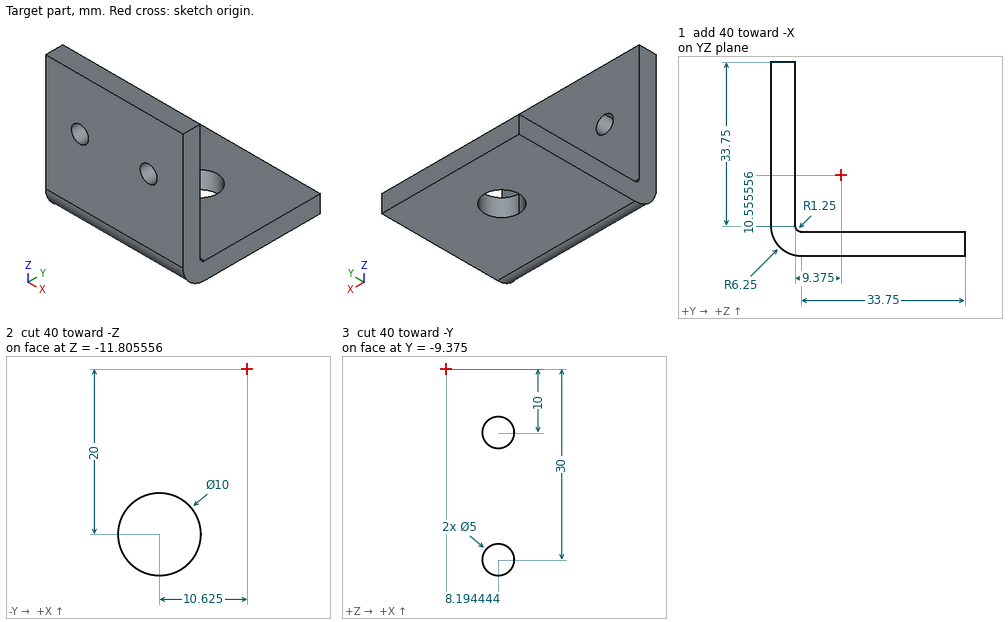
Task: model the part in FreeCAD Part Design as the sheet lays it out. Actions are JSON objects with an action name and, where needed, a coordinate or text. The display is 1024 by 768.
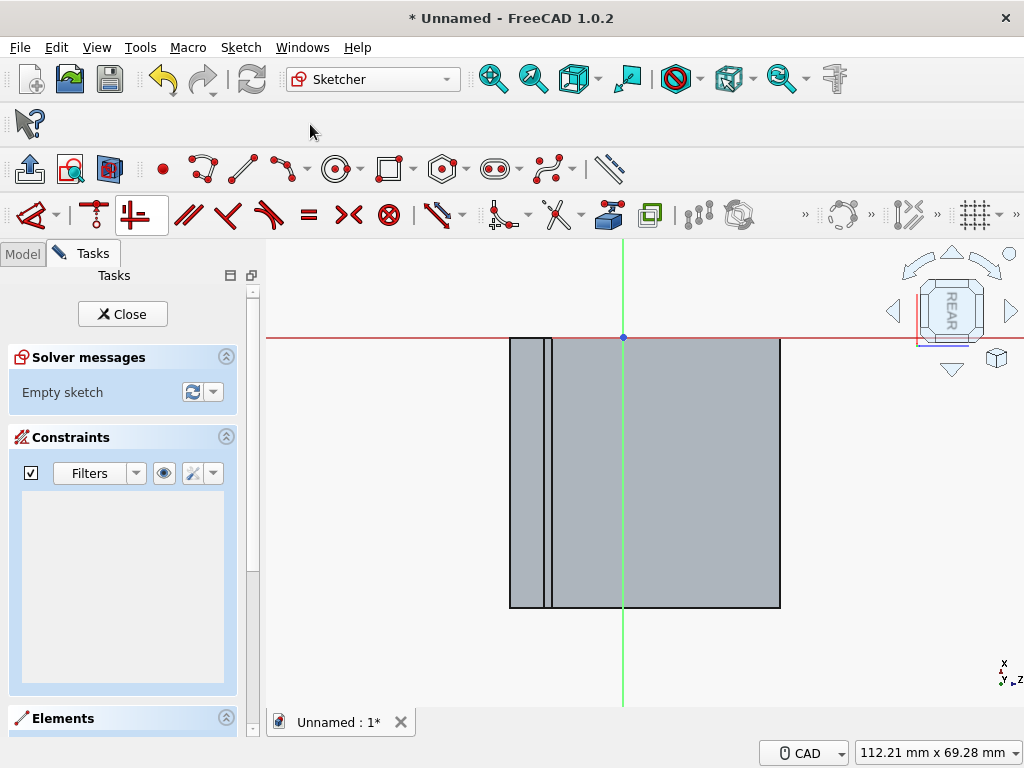
{"action": "key", "text": "q s"}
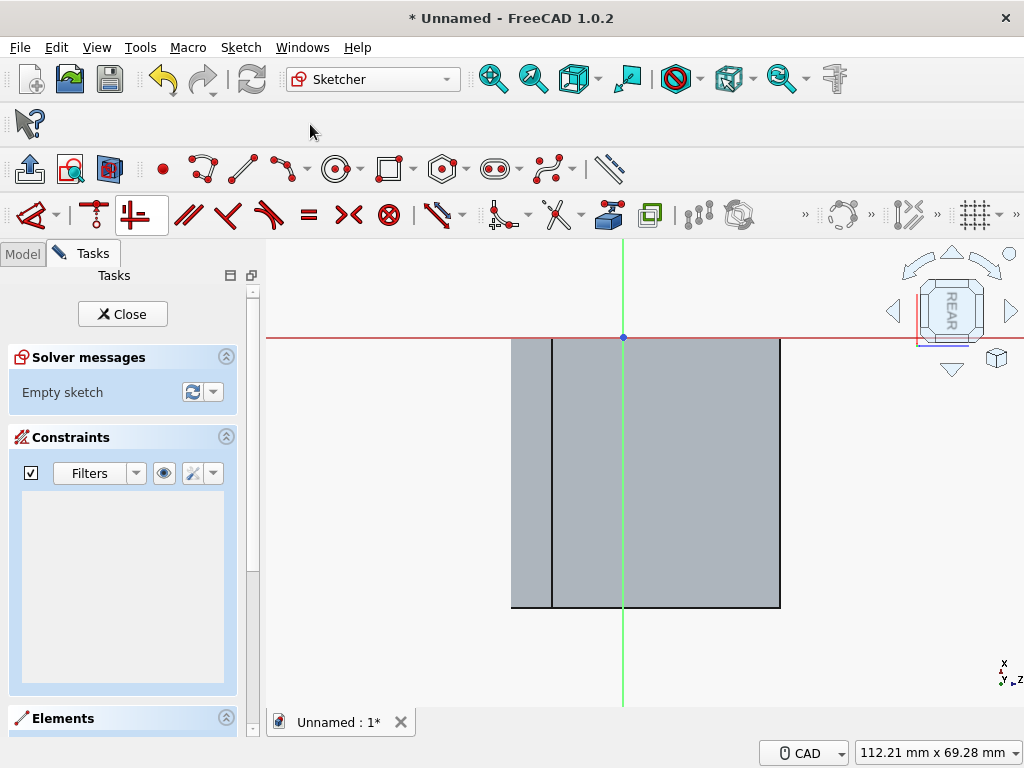
{"action": "left_click", "coordinate": [336, 170]}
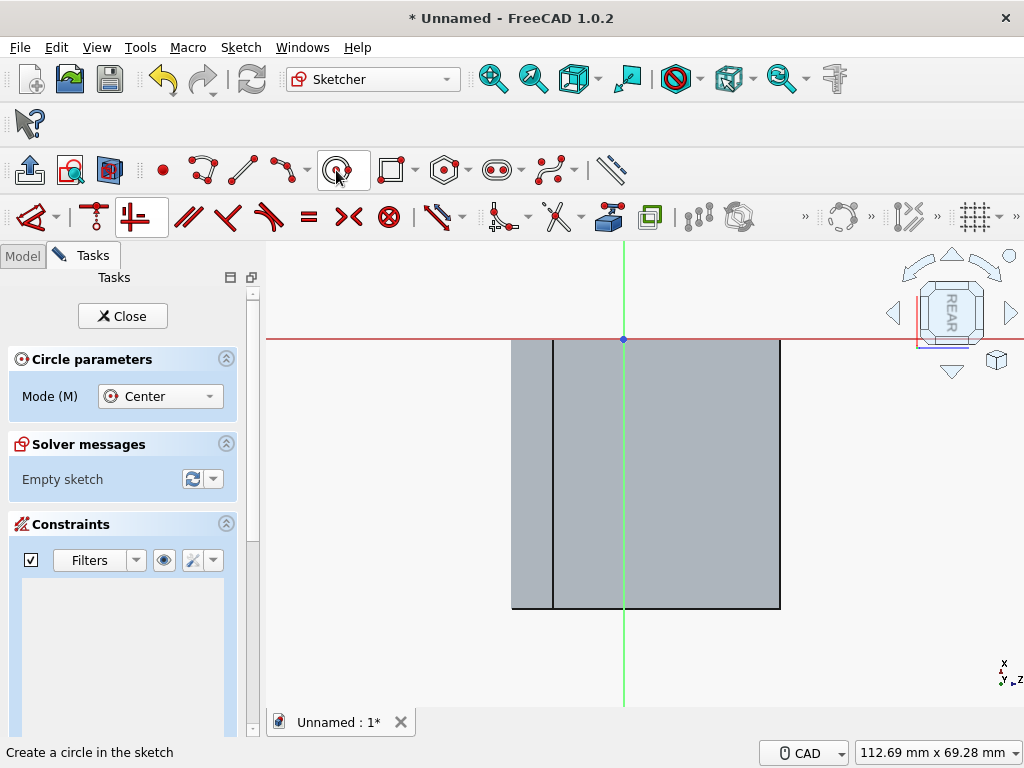
{"action": "scroll", "coordinate": [679, 541], "scroll_direction": "up", "scroll_amount": 2}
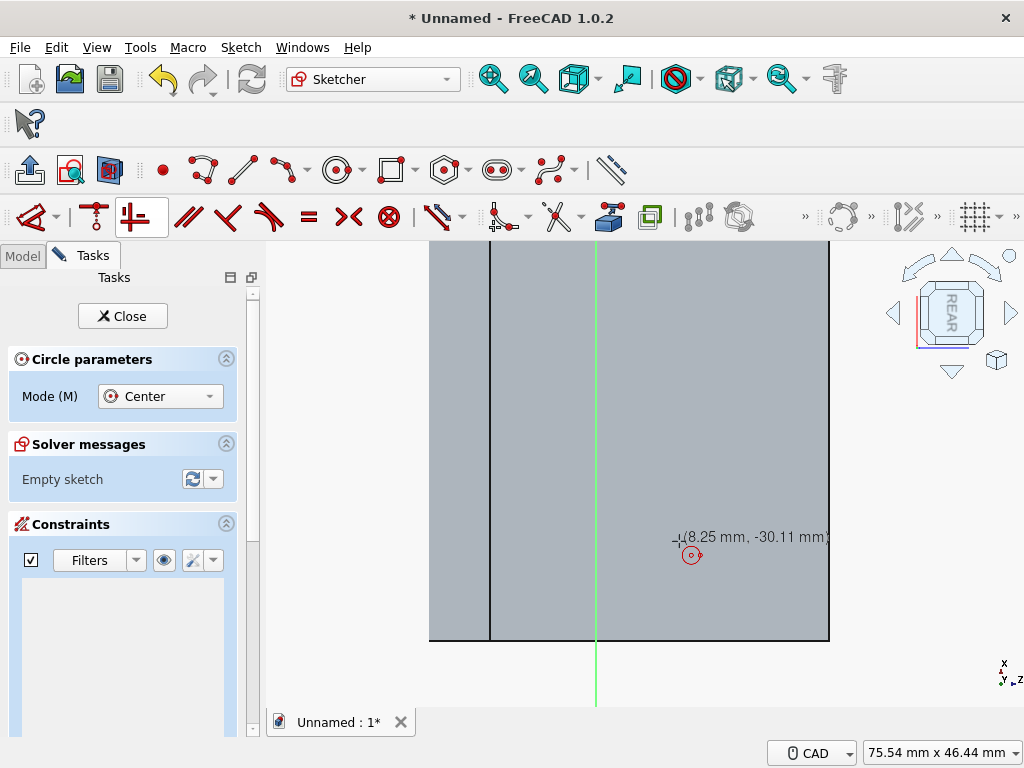
{"action": "left_click", "coordinate": [678, 541]}
{"action": "mouse_move", "coordinate": [696, 523]}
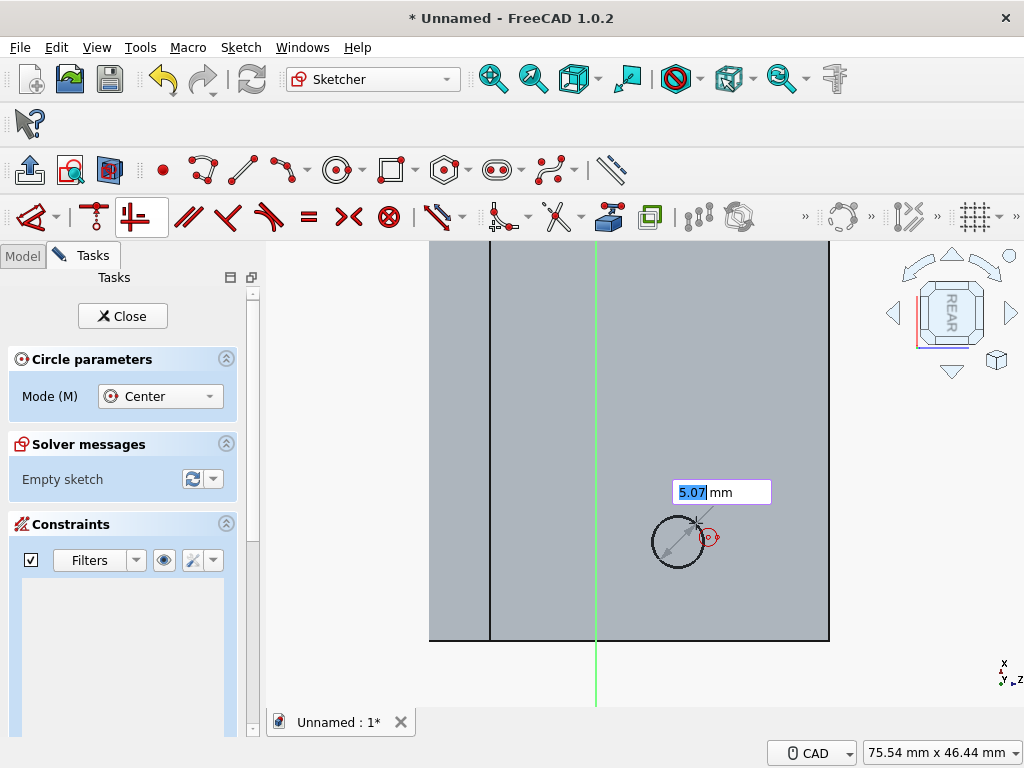
{"action": "type", "text": "5"}
{"action": "key", "text": "Return"}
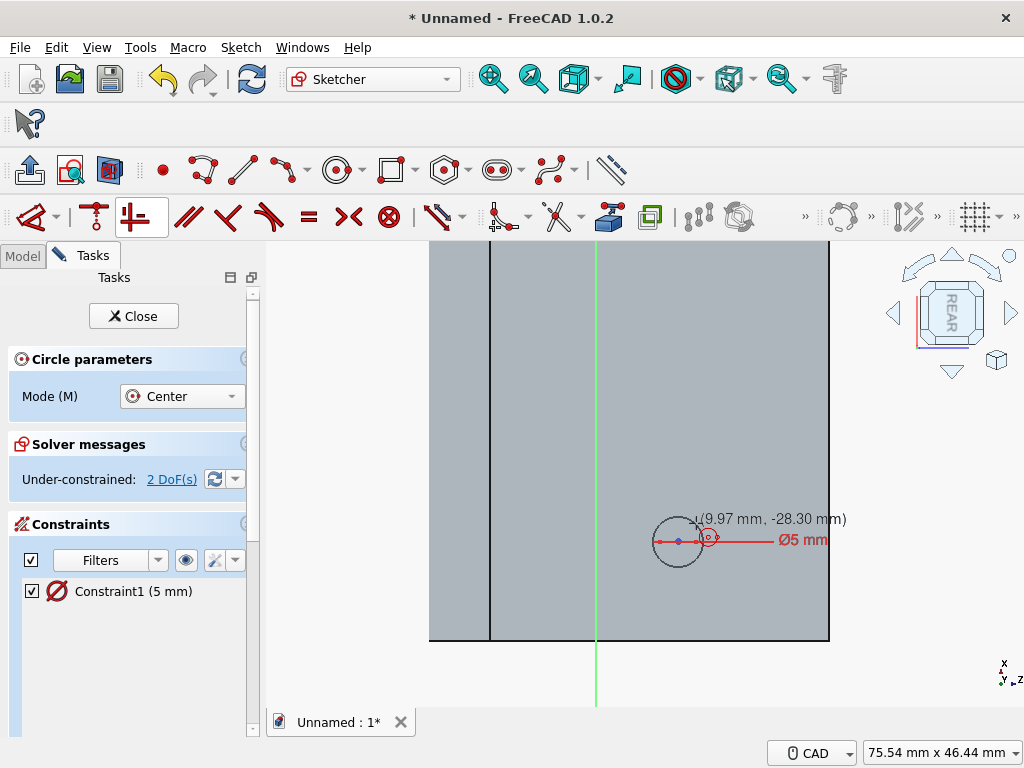
{"action": "left_click", "coordinate": [678, 340]}
{"action": "mouse_move", "coordinate": [696, 323]}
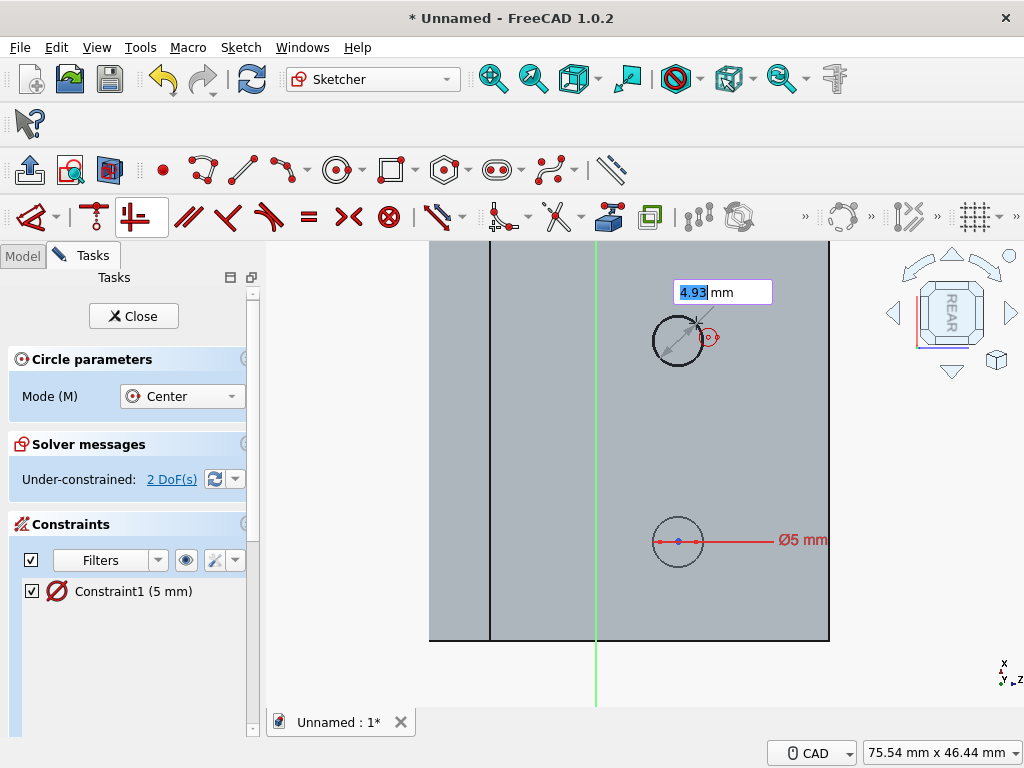
{"action": "type", "text": "5"}
{"action": "key", "text": "Return"}
{"action": "key", "text": "Escape"}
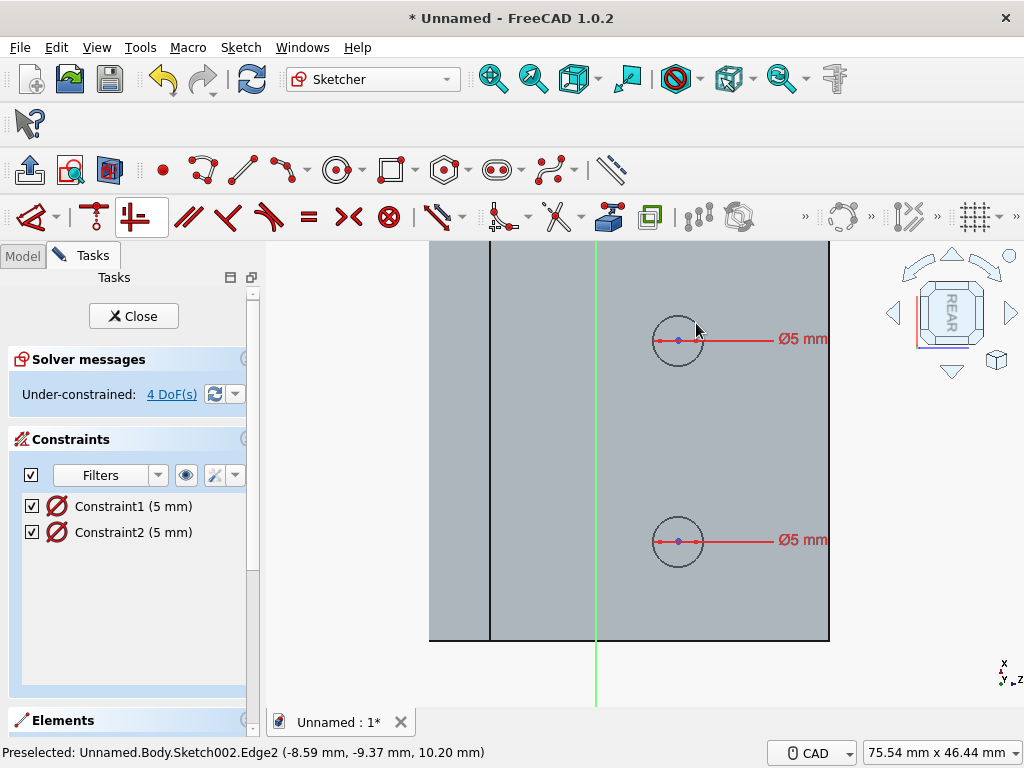
{"action": "left_click", "coordinate": [678, 542]}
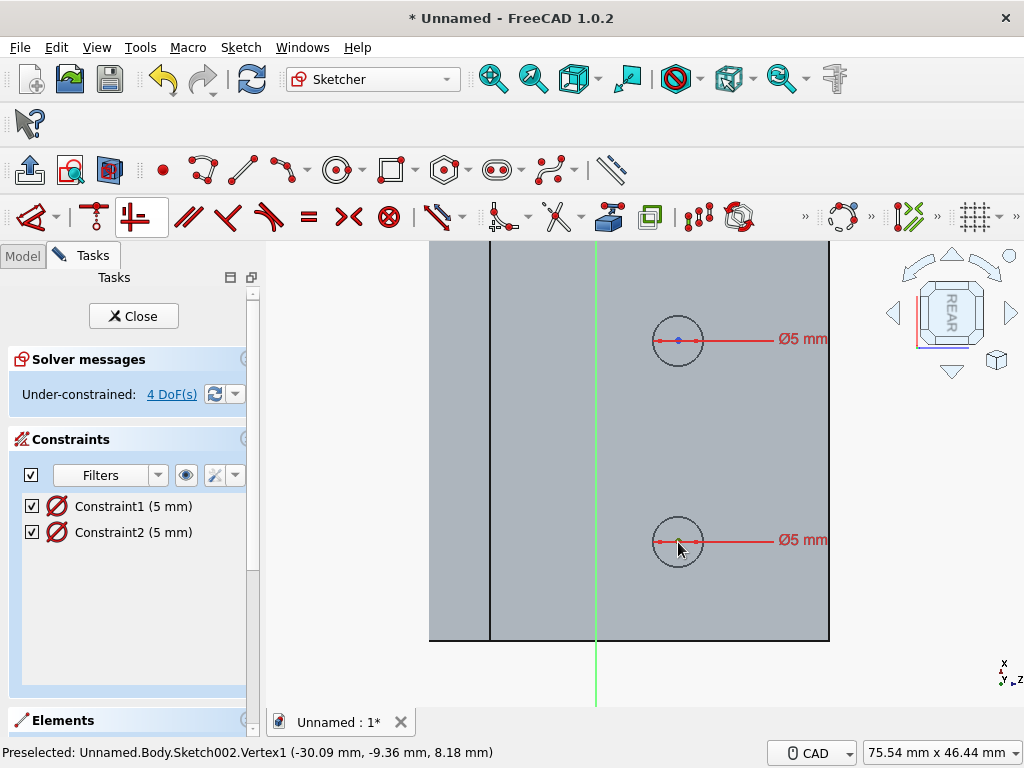
{"action": "left_click", "coordinate": [678, 341]}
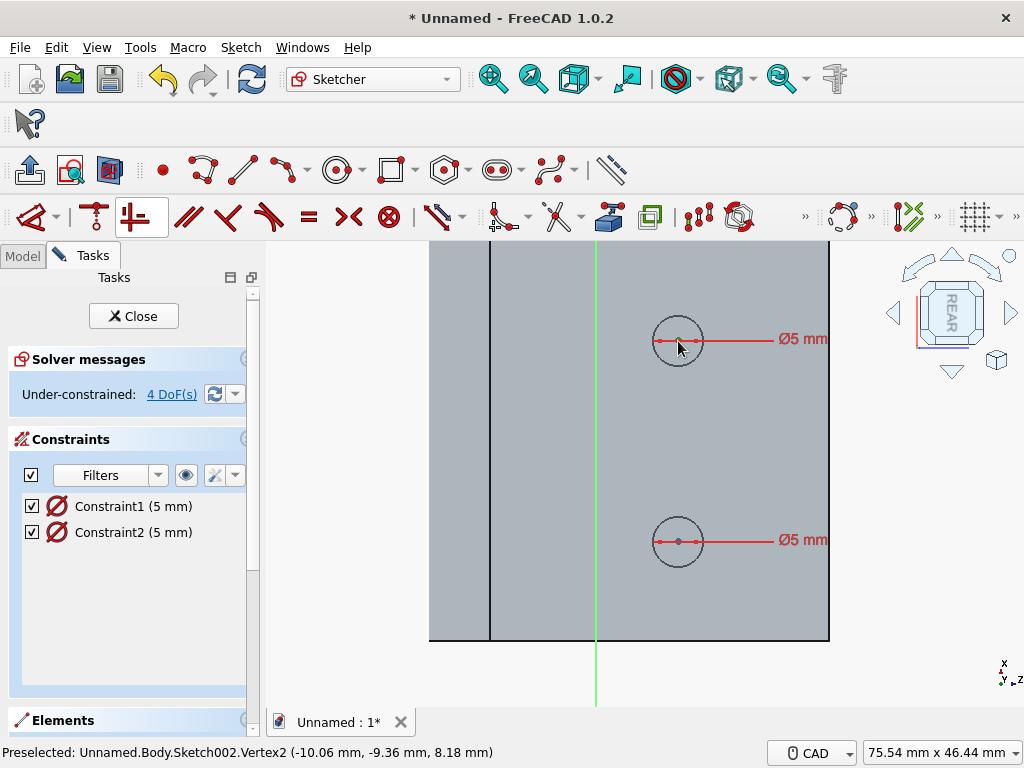
{"action": "key", "text": "v"}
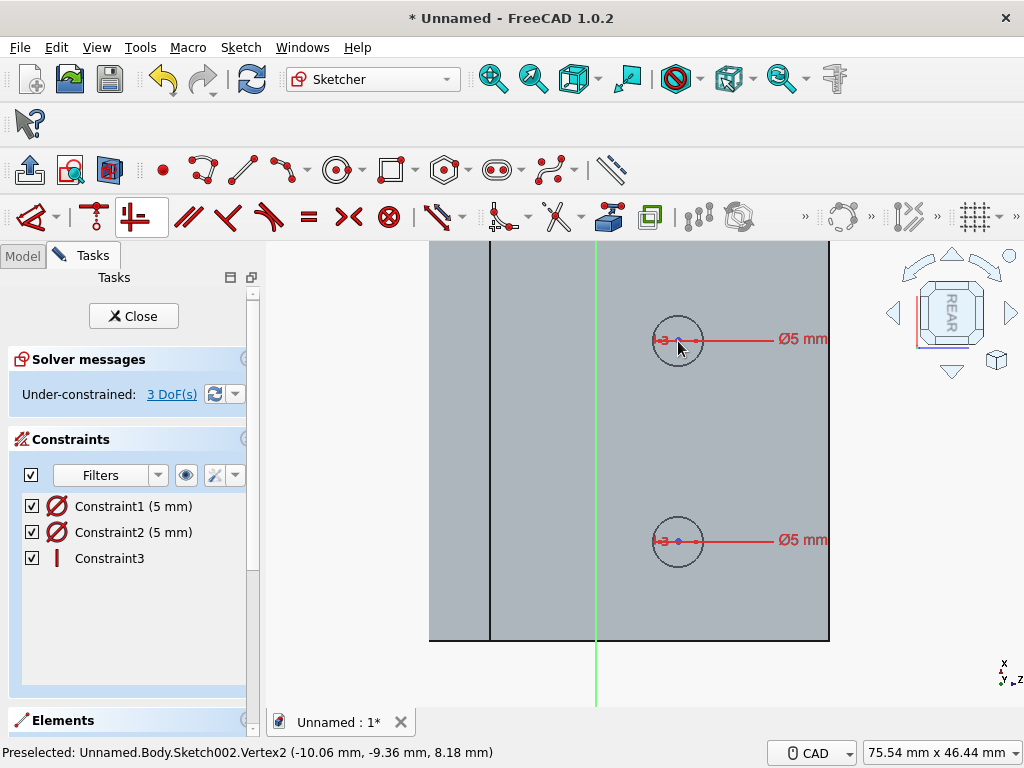
{"action": "left_click", "coordinate": [32, 218]}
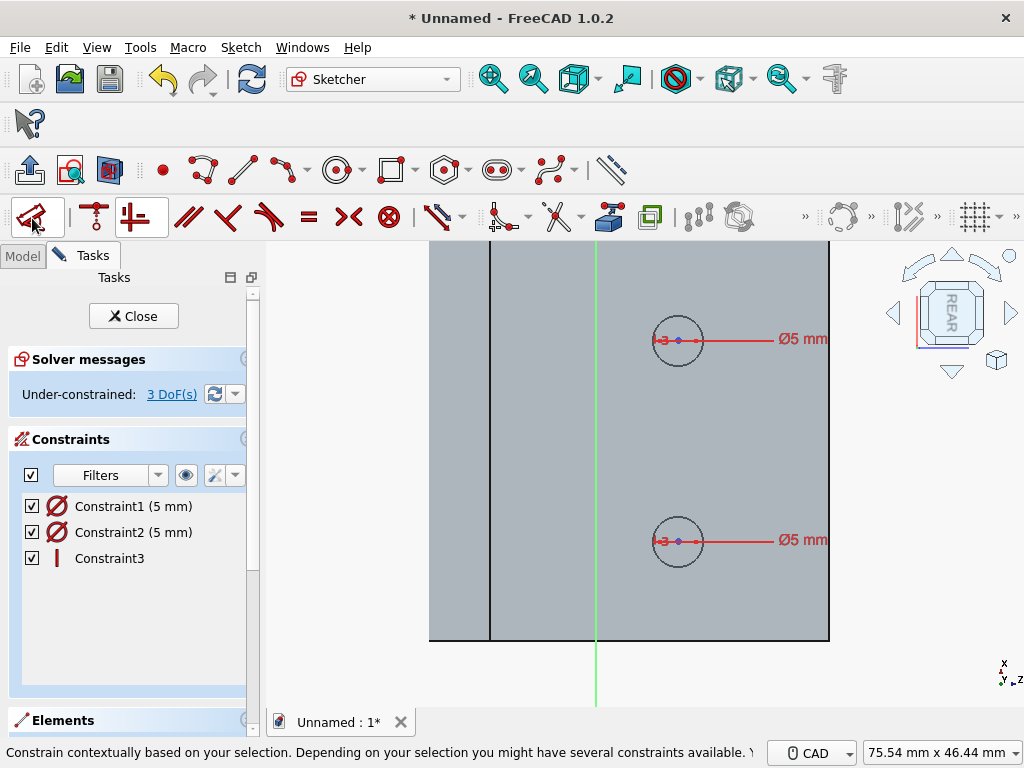
{"action": "left_click", "coordinate": [678, 542]}
{"action": "left_click", "coordinate": [562, 406]}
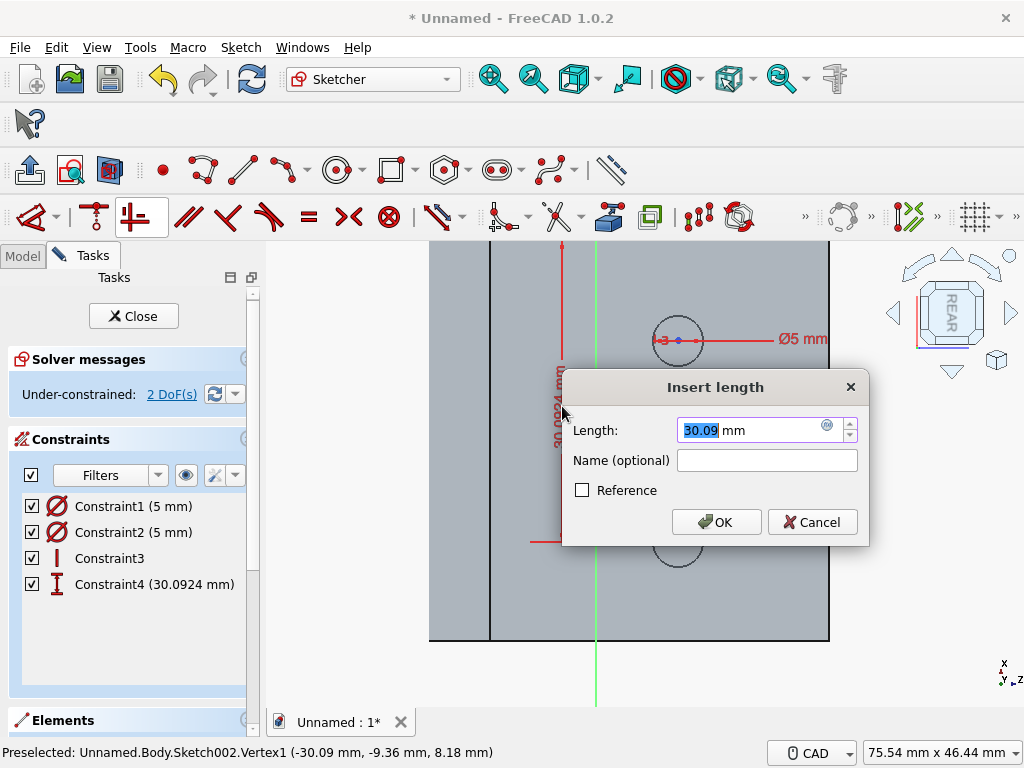
{"action": "type", "text": "30"}
{"action": "key", "text": "Return"}